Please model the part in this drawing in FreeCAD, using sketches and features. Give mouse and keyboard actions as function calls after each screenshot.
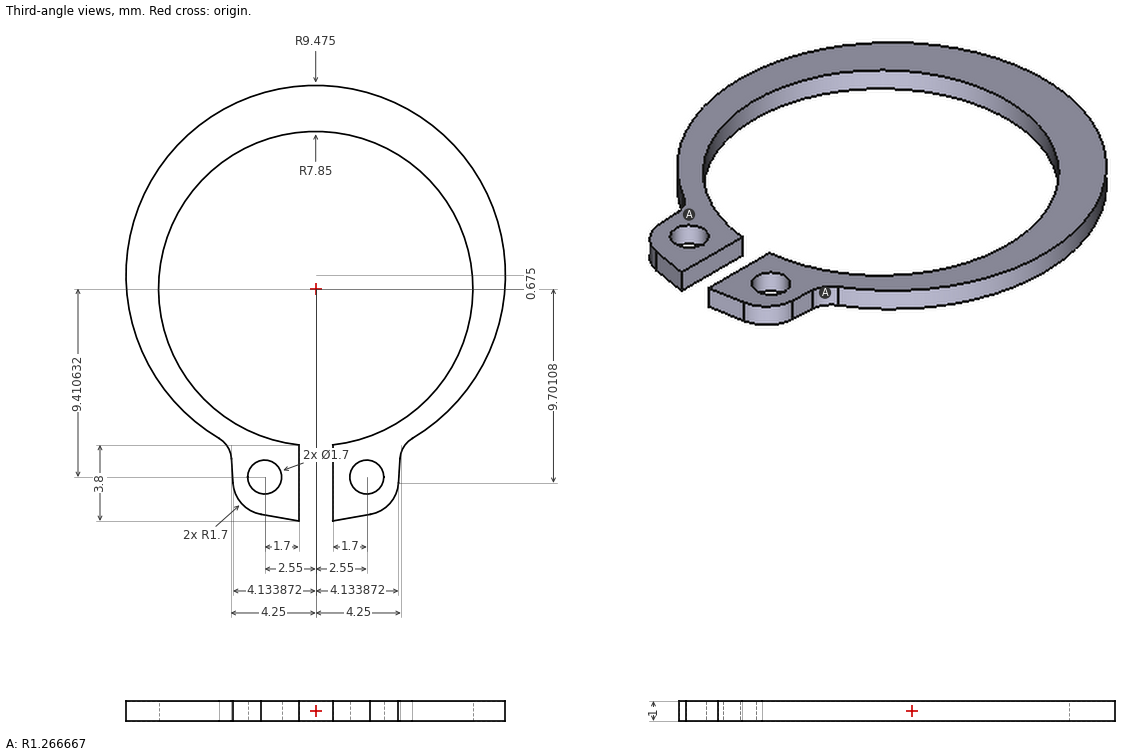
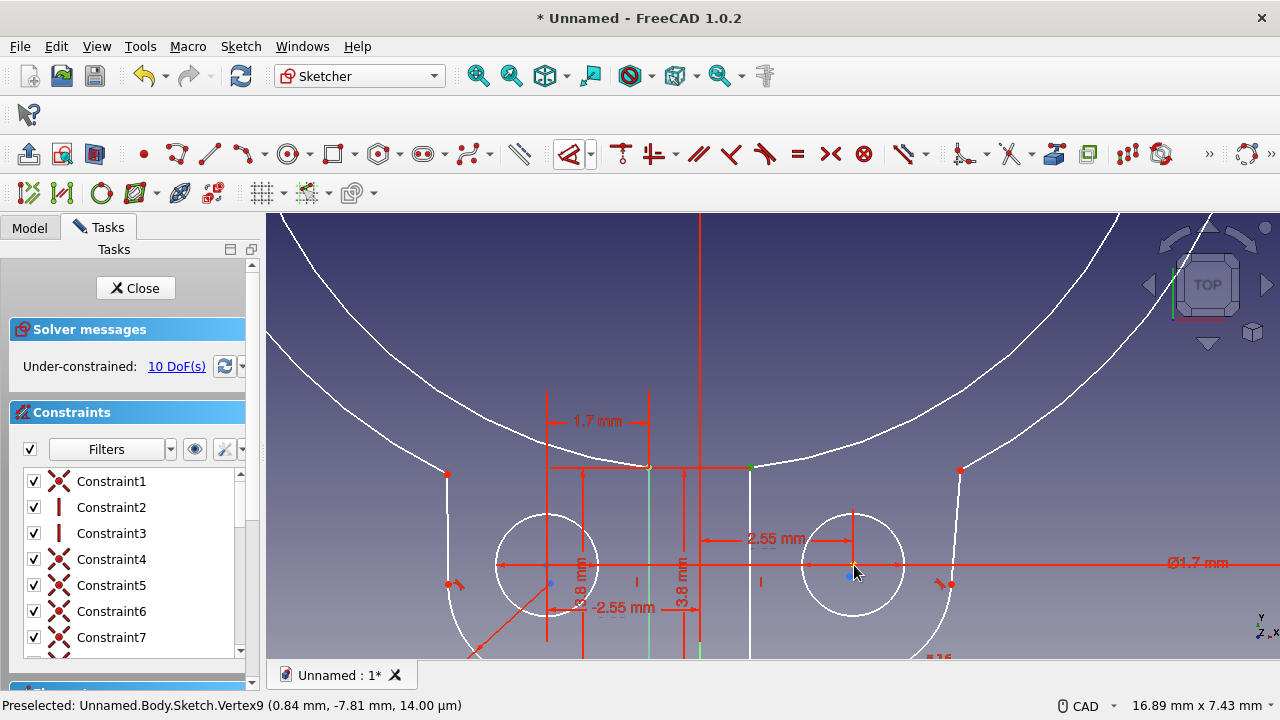
click(853, 565)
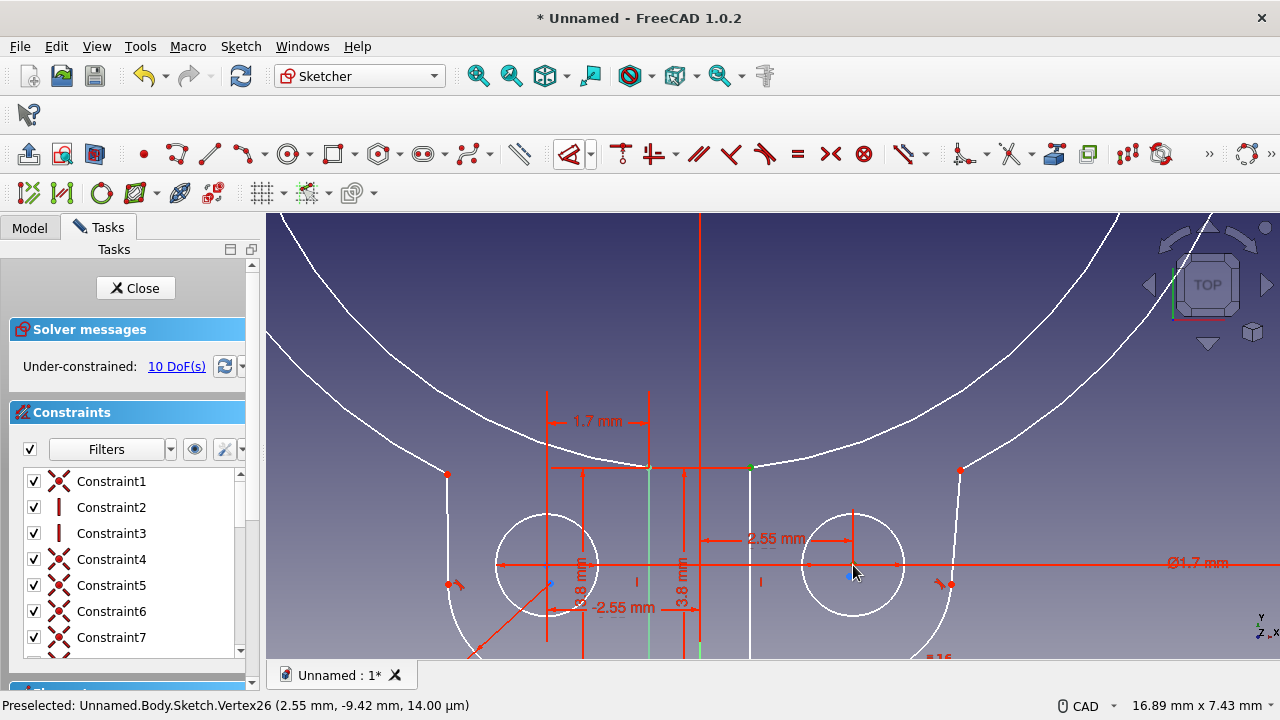
click(590, 154)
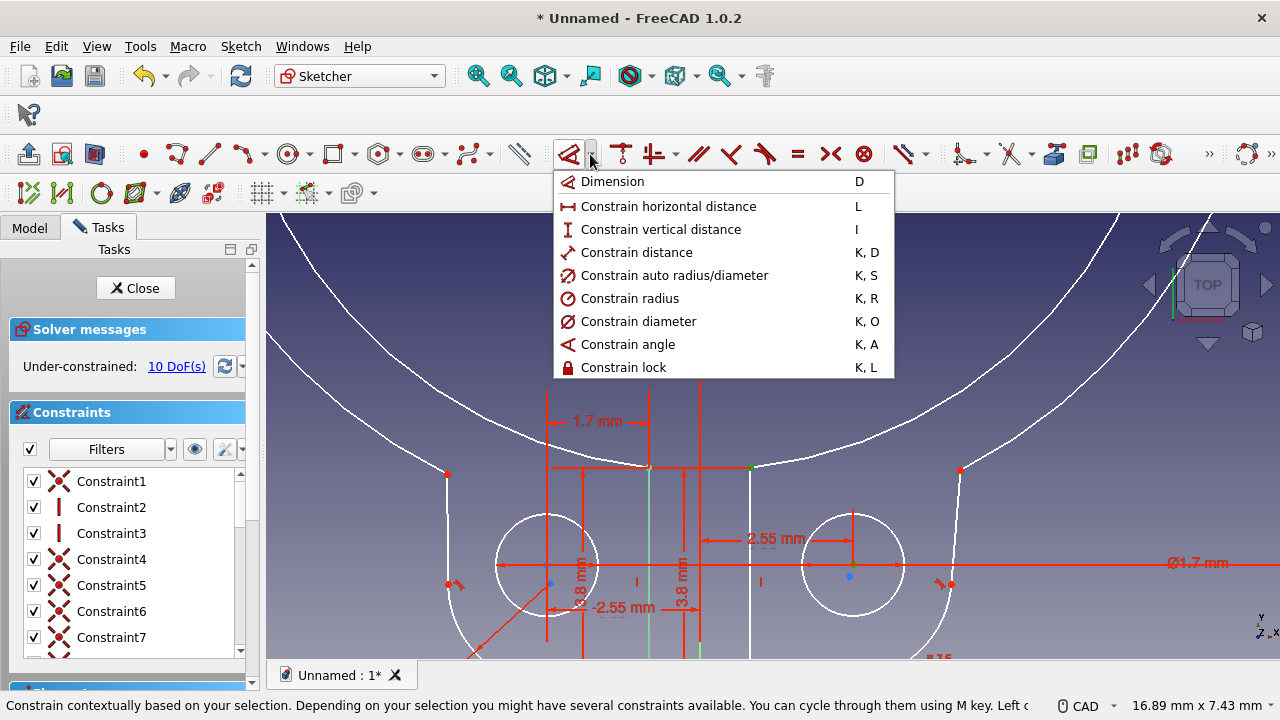
click(724, 206)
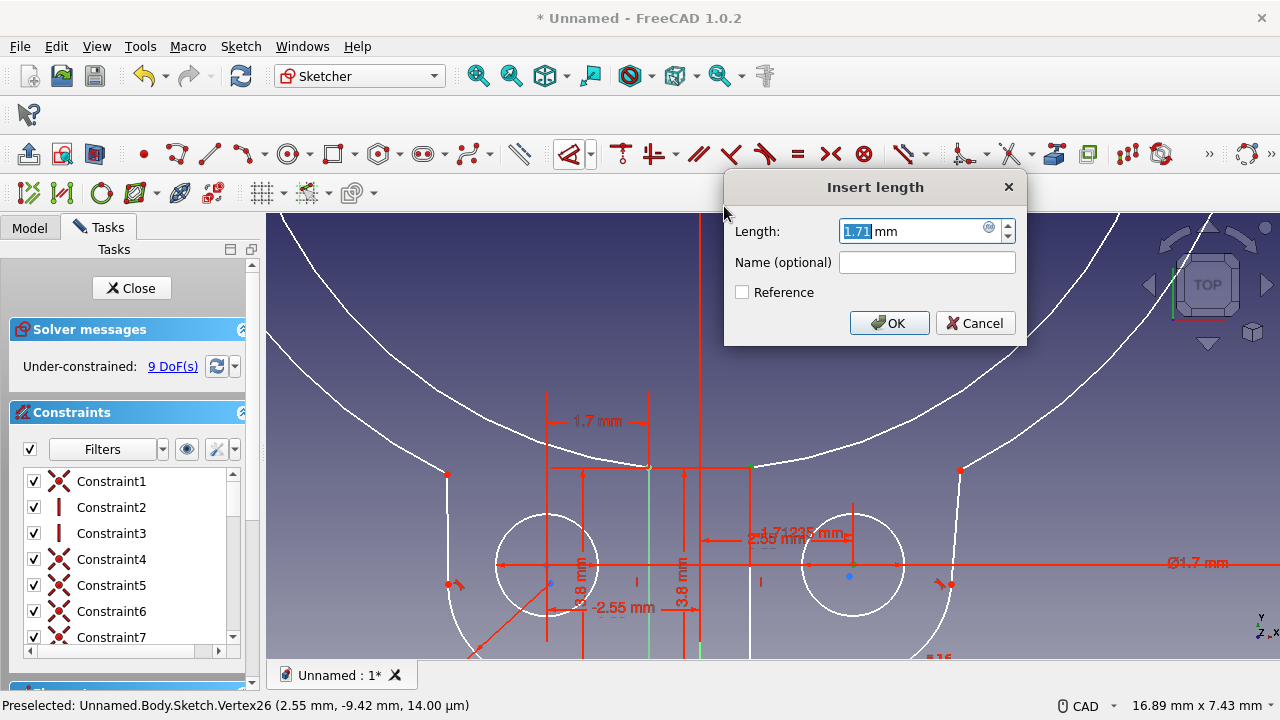
text(1.7)
key(Return)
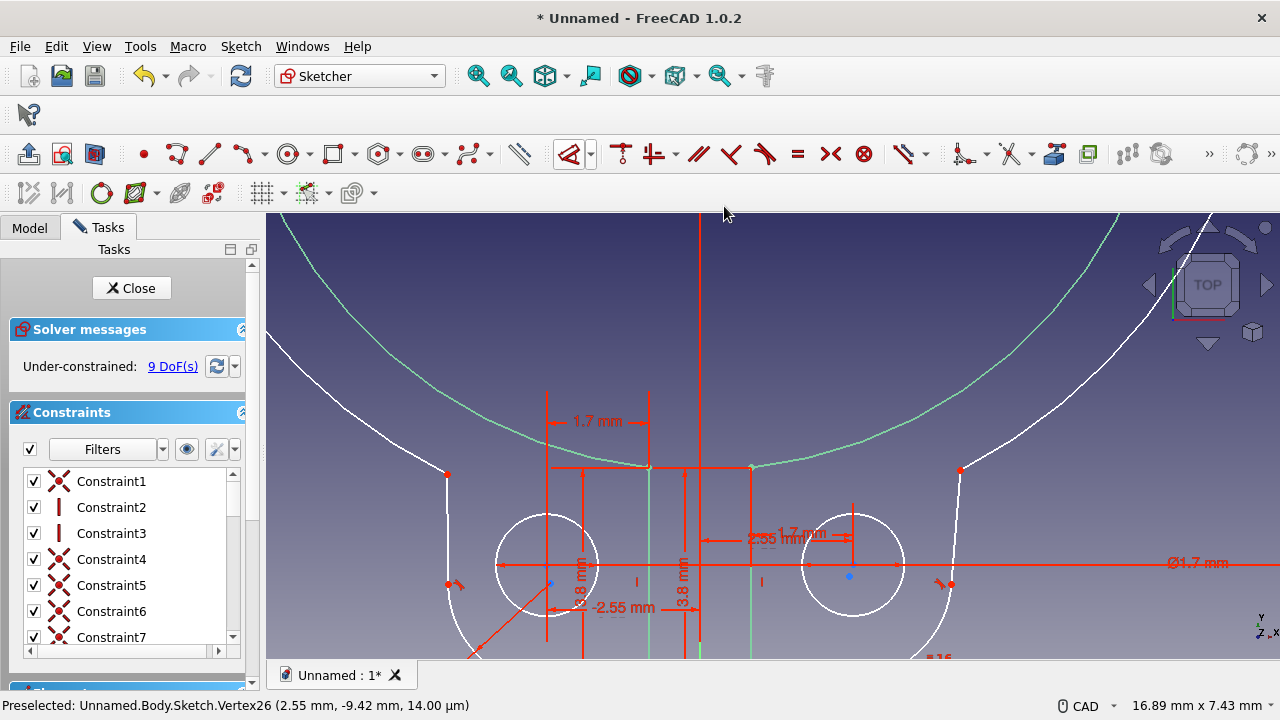
scroll(706, 535, down, 8)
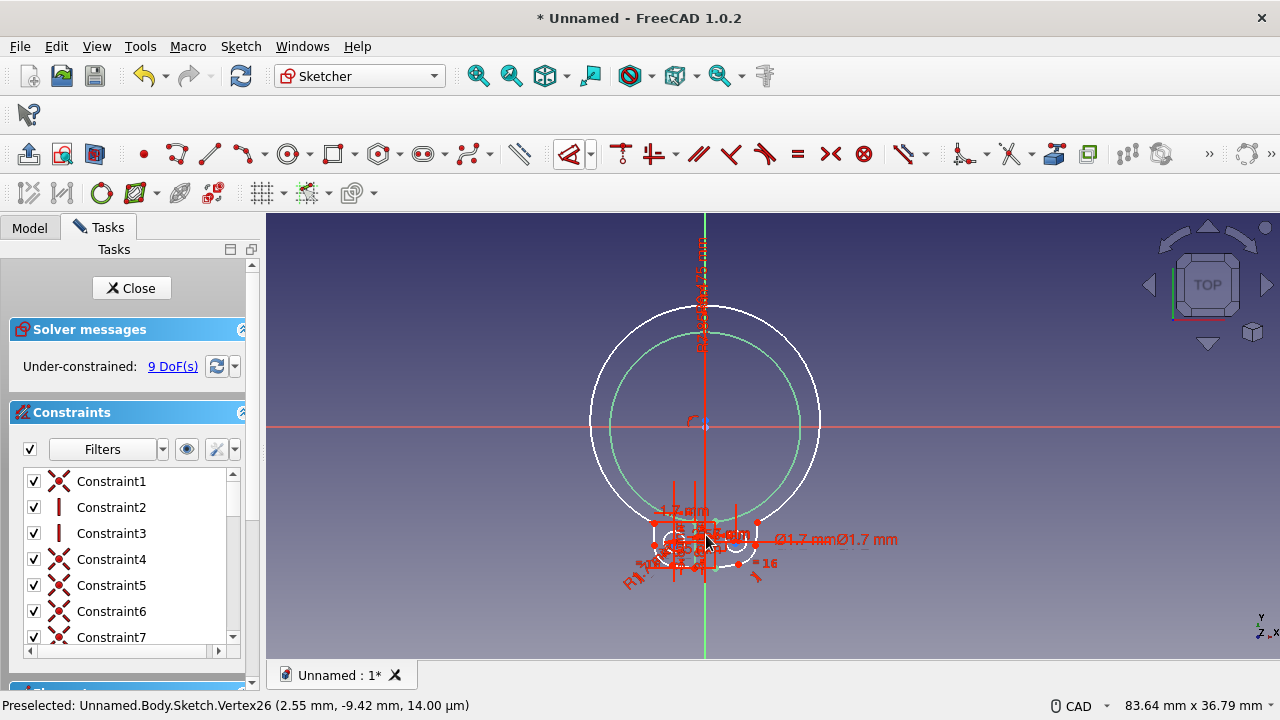
click(758, 522)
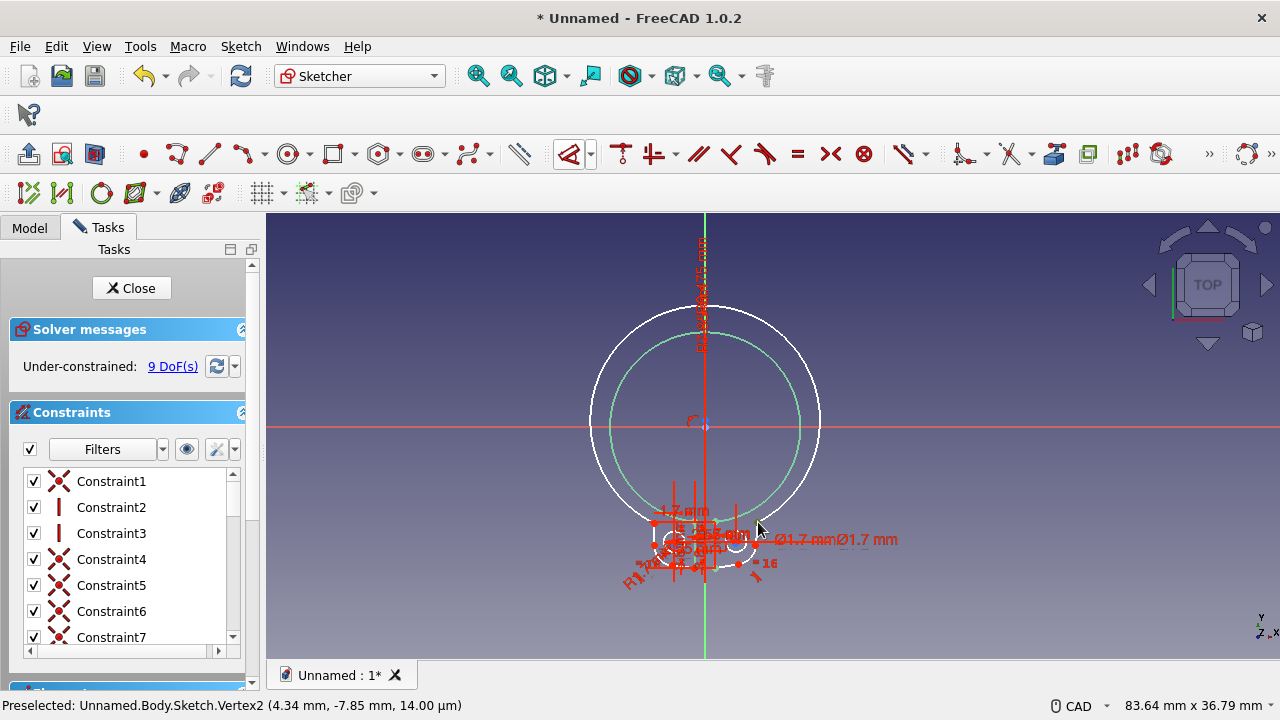
click(590, 154)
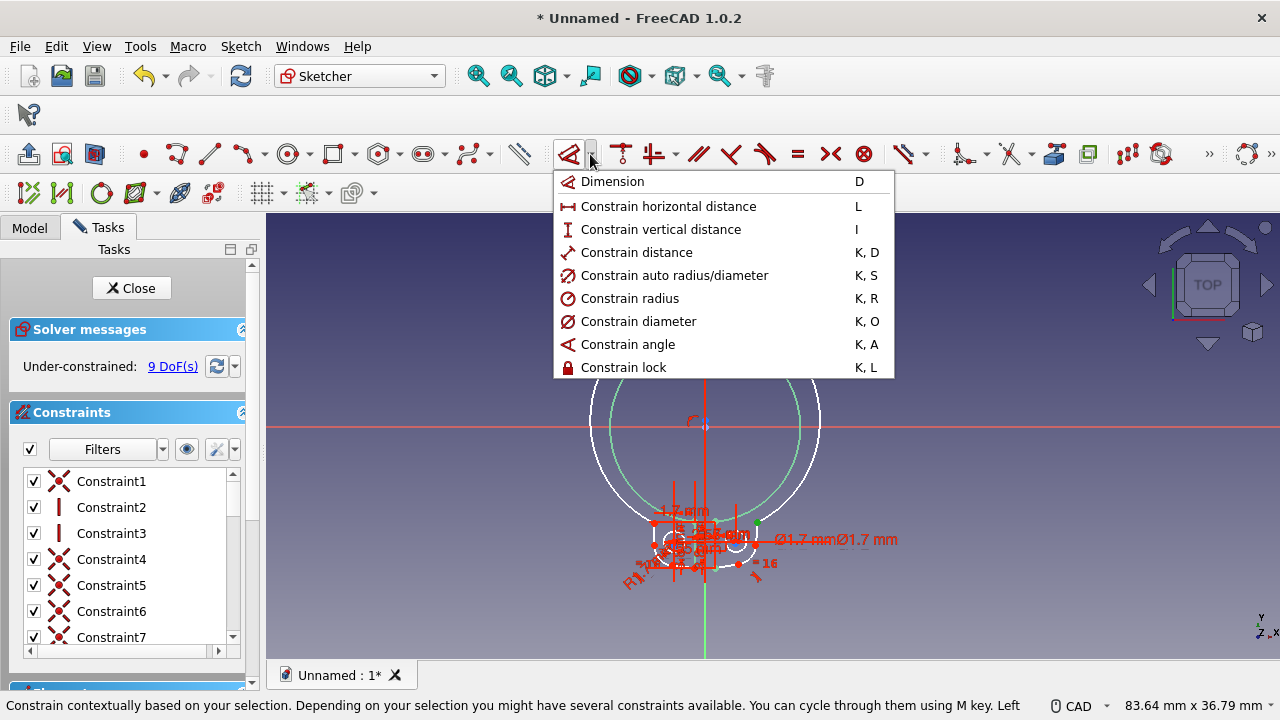
click(724, 206)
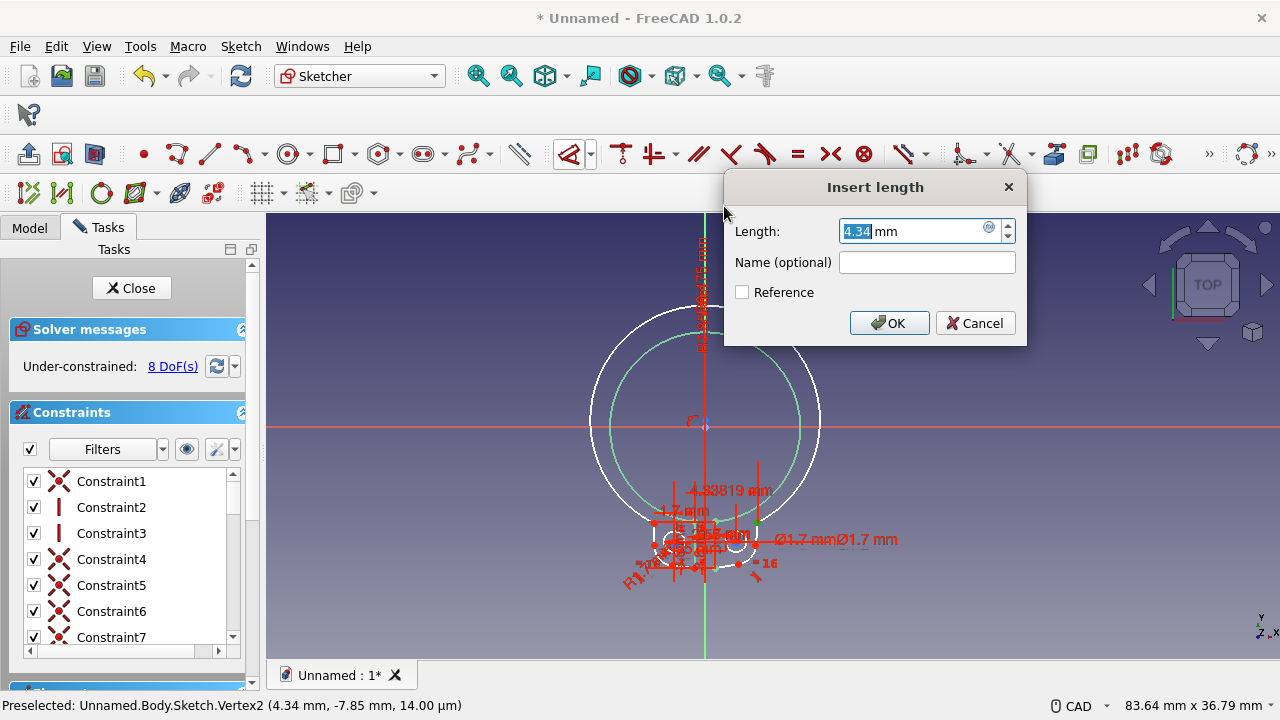
text(4.25)
key(Return)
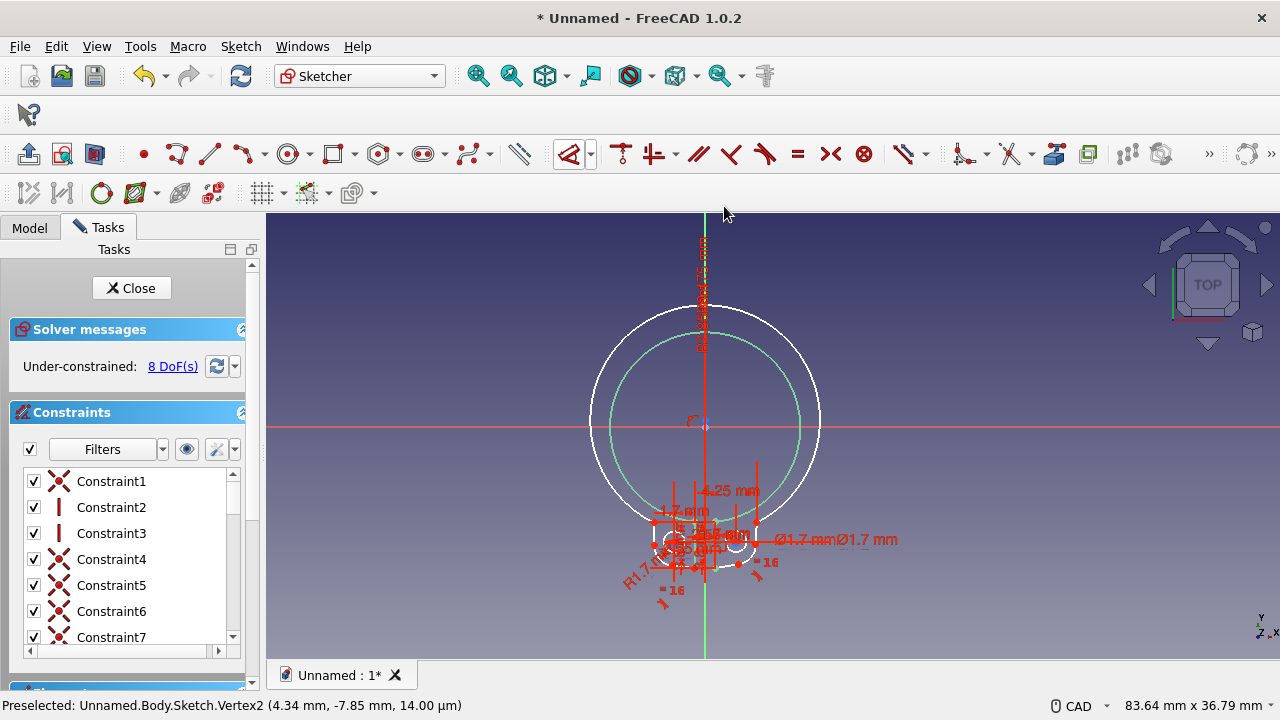
click(654, 523)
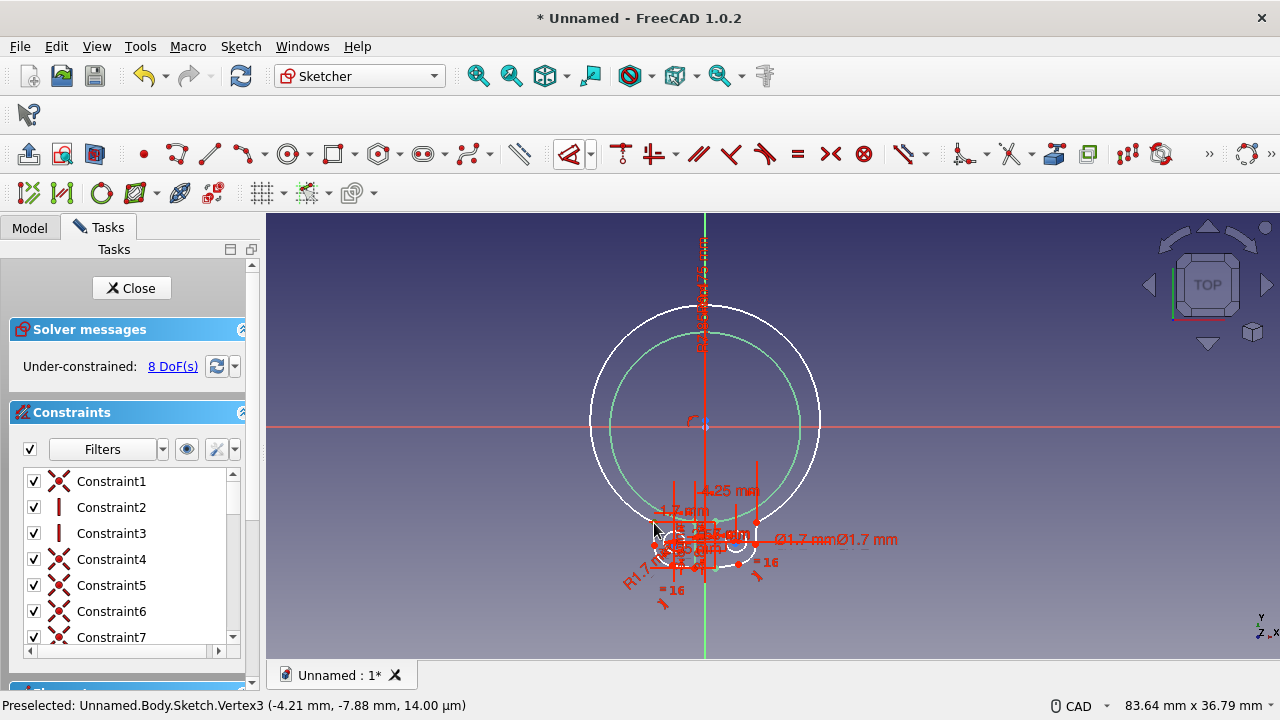
key(l)